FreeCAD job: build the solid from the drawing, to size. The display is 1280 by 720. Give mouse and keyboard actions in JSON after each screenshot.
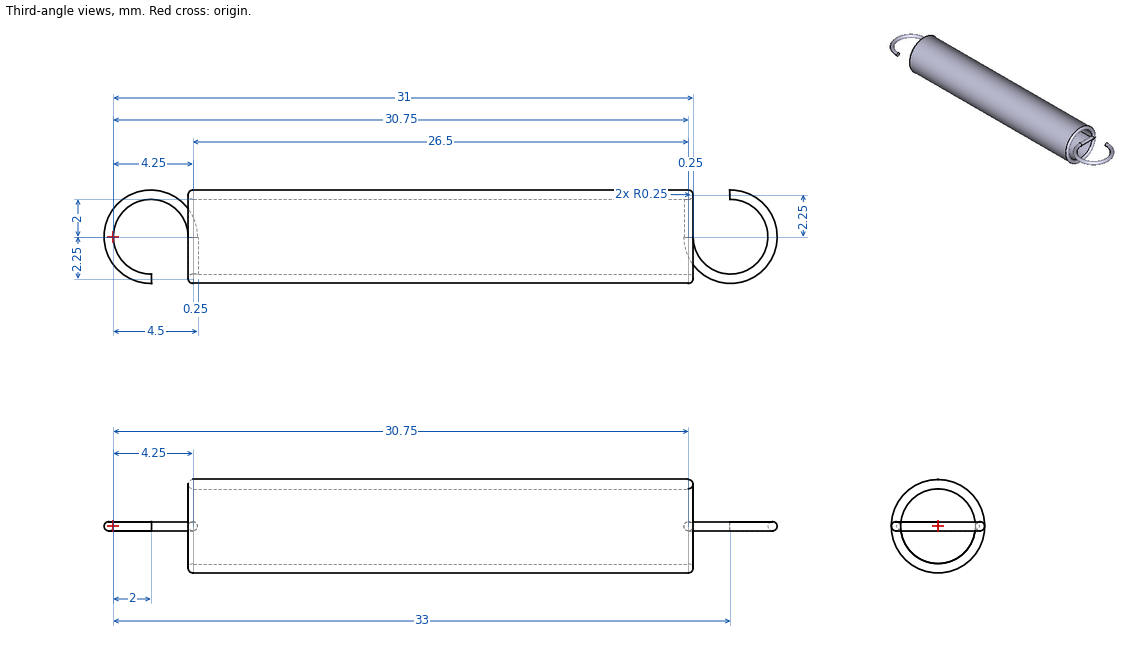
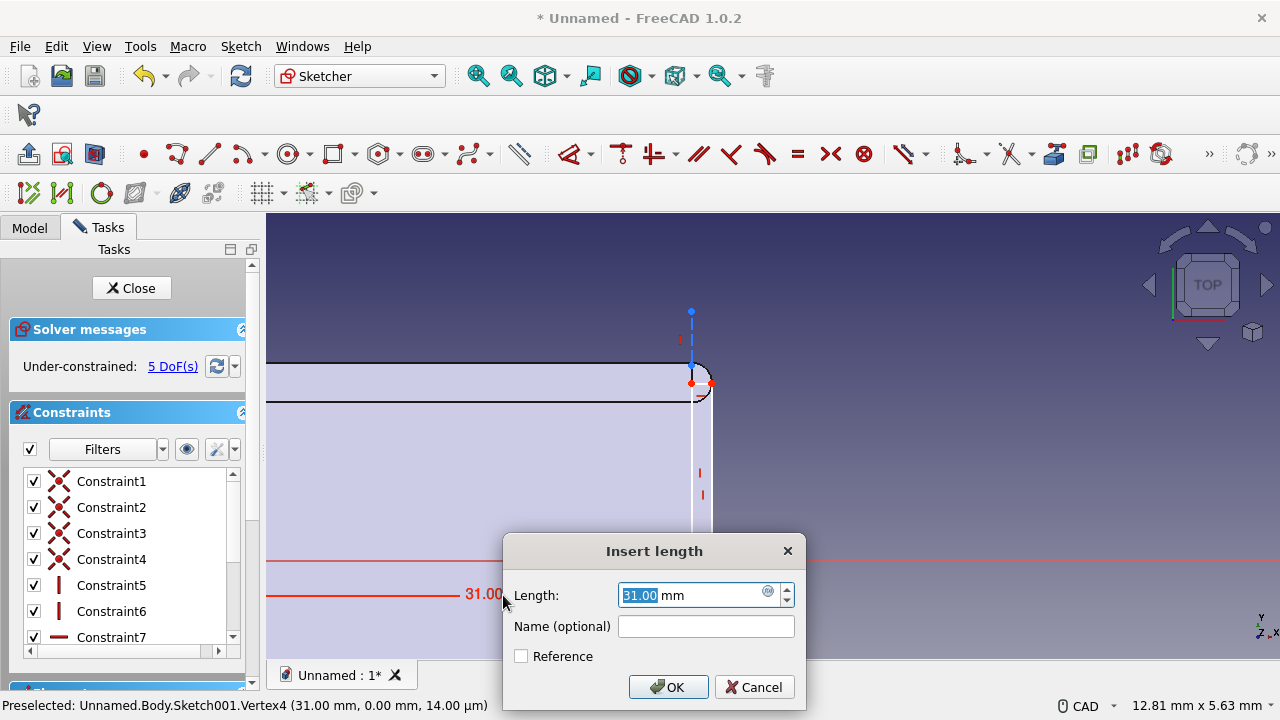
{"action": "type", "text": "31"}
{"action": "key", "text": "Return"}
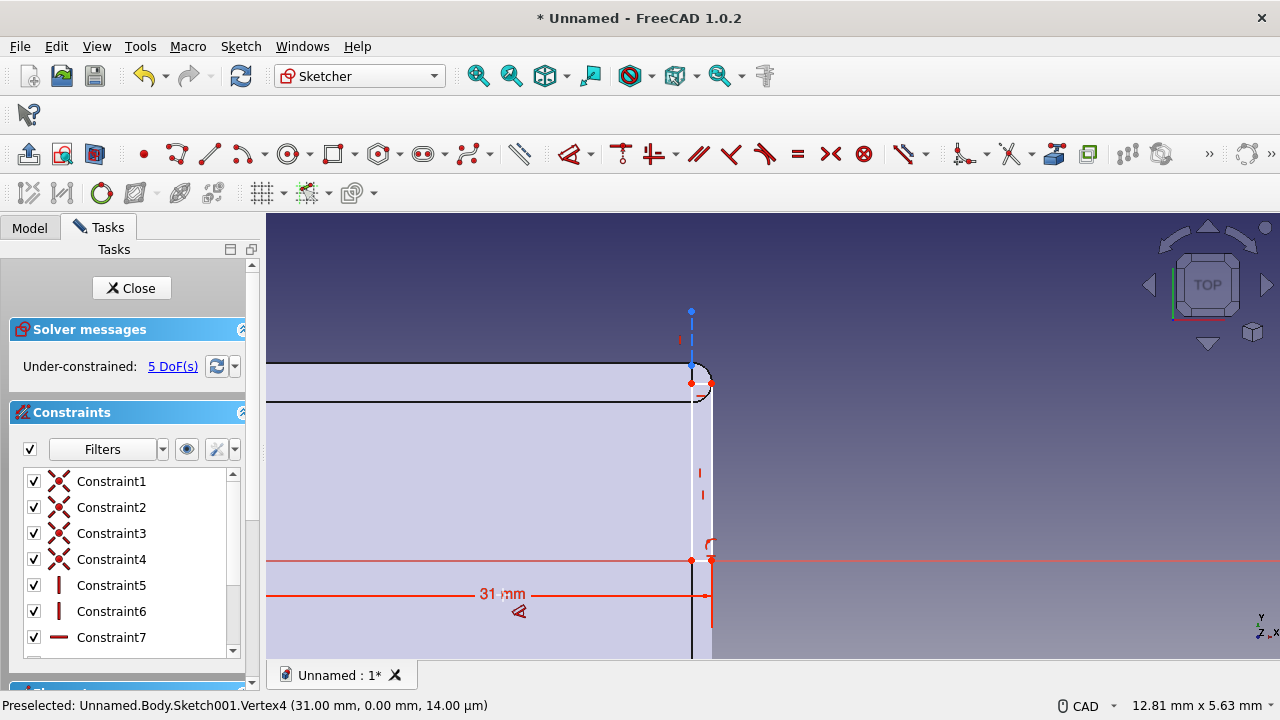
{"action": "left_click", "coordinate": [692, 437]}
{"action": "left_click", "coordinate": [658, 472]}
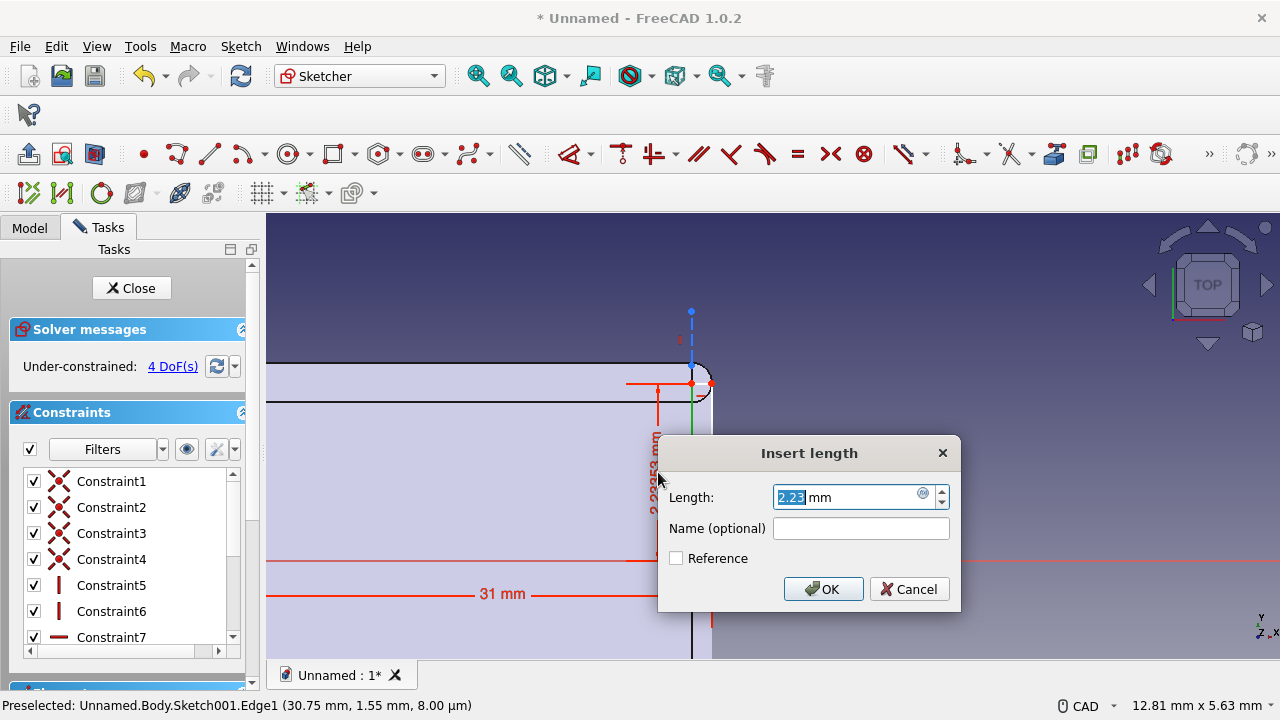
{"action": "type", "text": "2.25"}
{"action": "key", "text": "Return"}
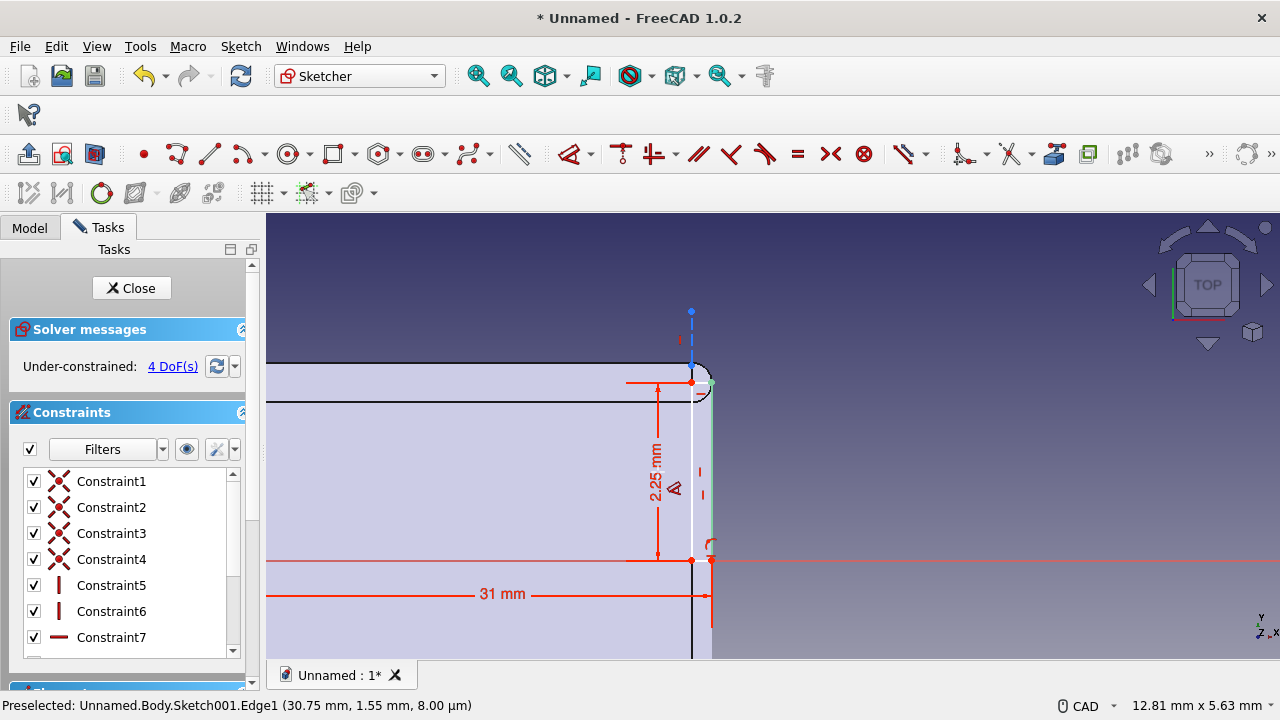
{"action": "scroll", "coordinate": [702, 561], "scroll_direction": "up", "scroll_amount": 4}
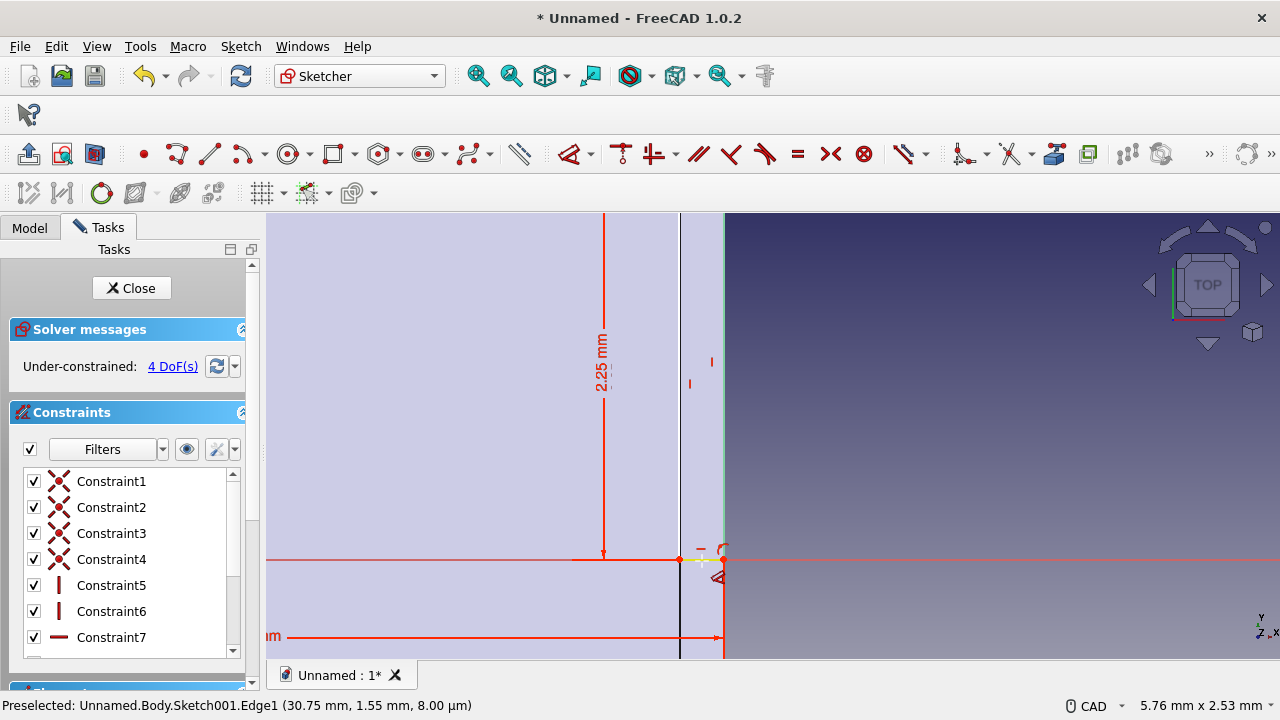
{"action": "left_click", "coordinate": [701, 560]}
{"action": "left_click", "coordinate": [701, 594]}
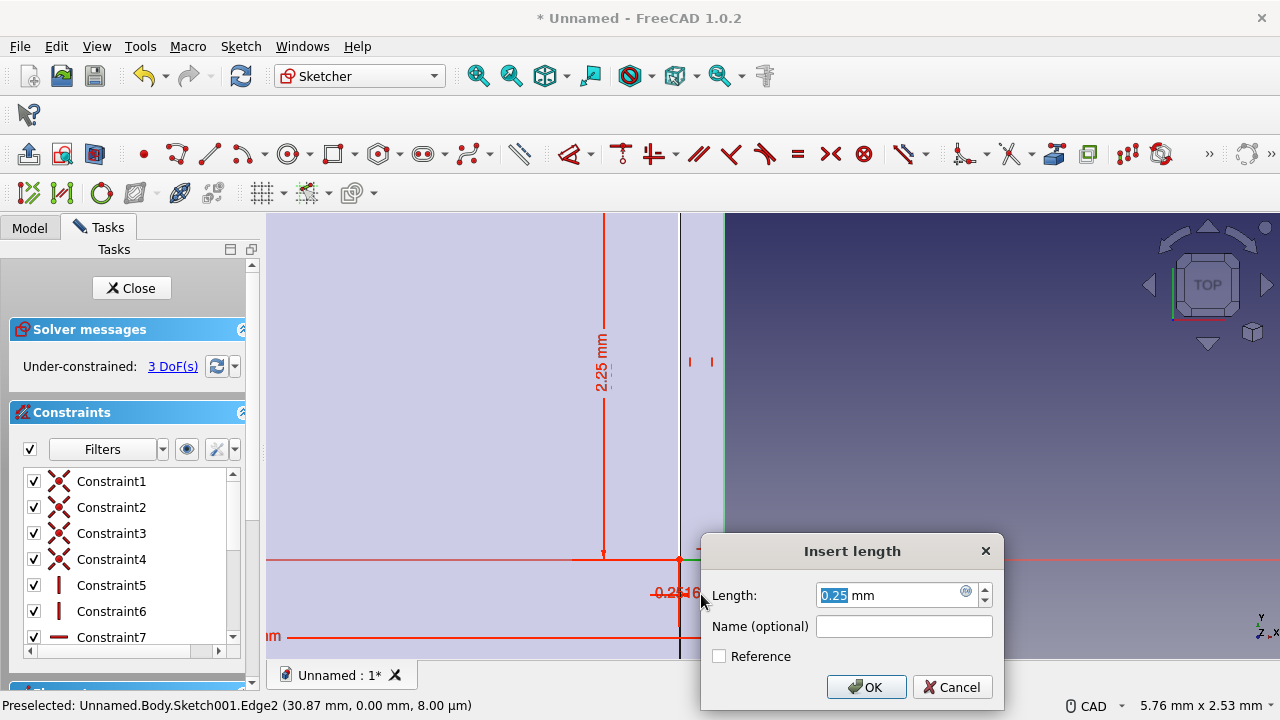
{"action": "type", "text": "0.25"}
{"action": "key", "text": "Return"}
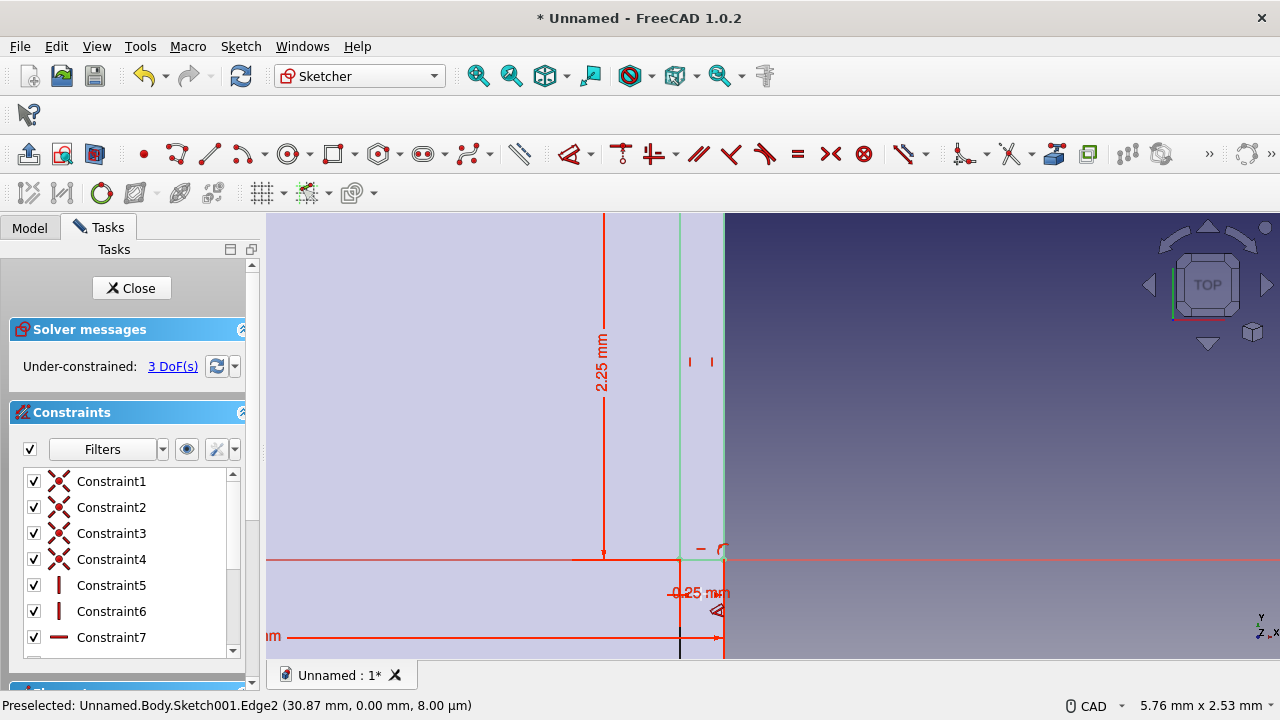
{"action": "scroll", "coordinate": [707, 562], "scroll_direction": "down", "scroll_amount": 4}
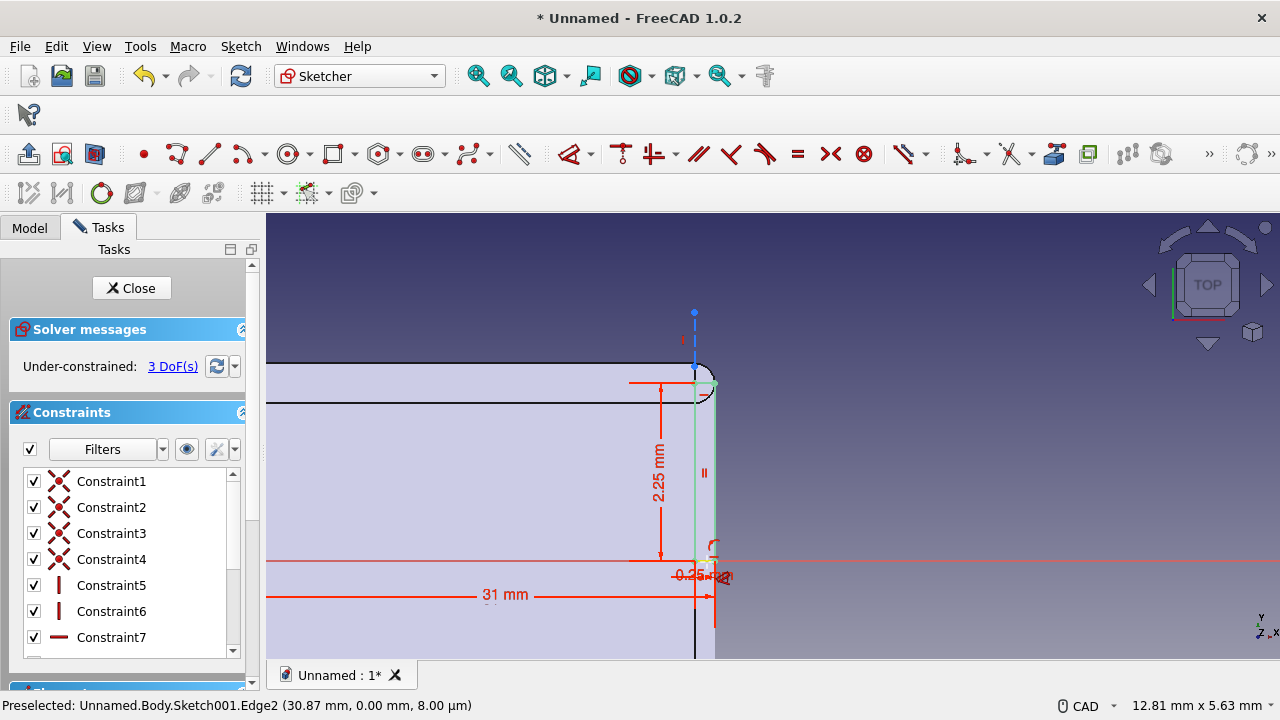
{"action": "left_click", "coordinate": [695, 367]}
{"action": "left_click", "coordinate": [402, 595]}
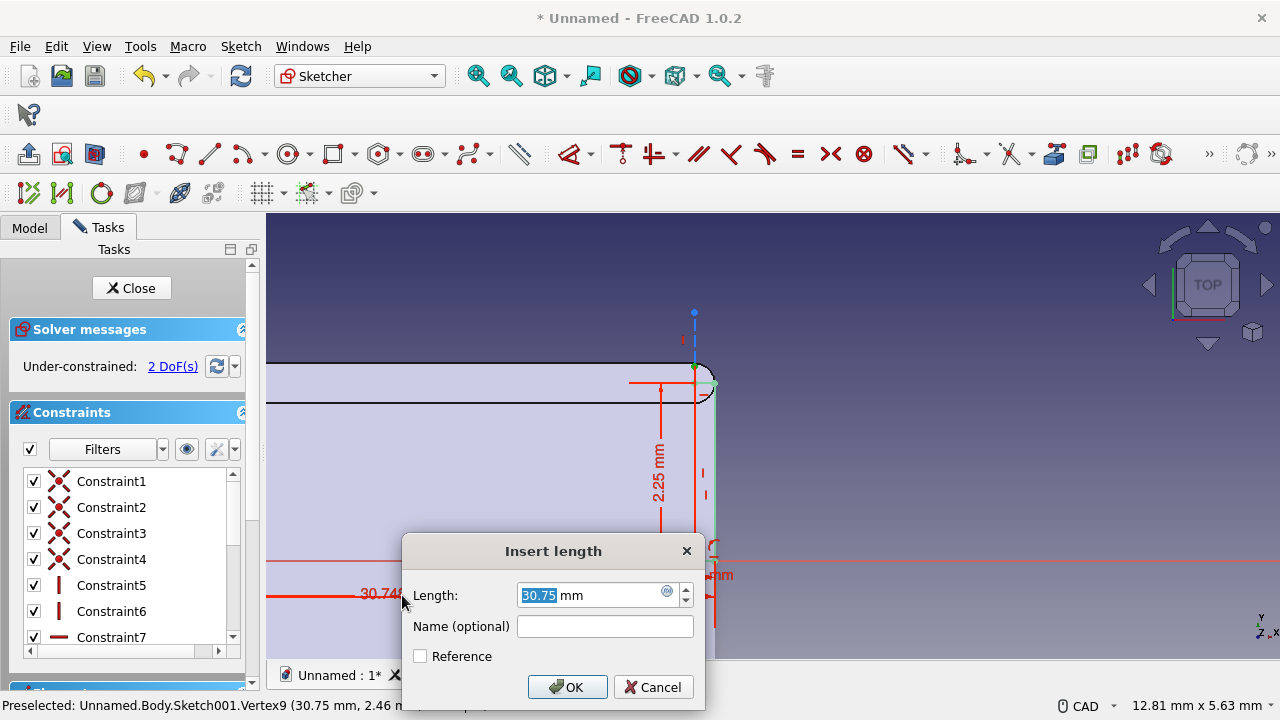
{"action": "type", "text": "30.75"}
{"action": "key", "text": "Return"}
{"action": "key", "text": "Escape"}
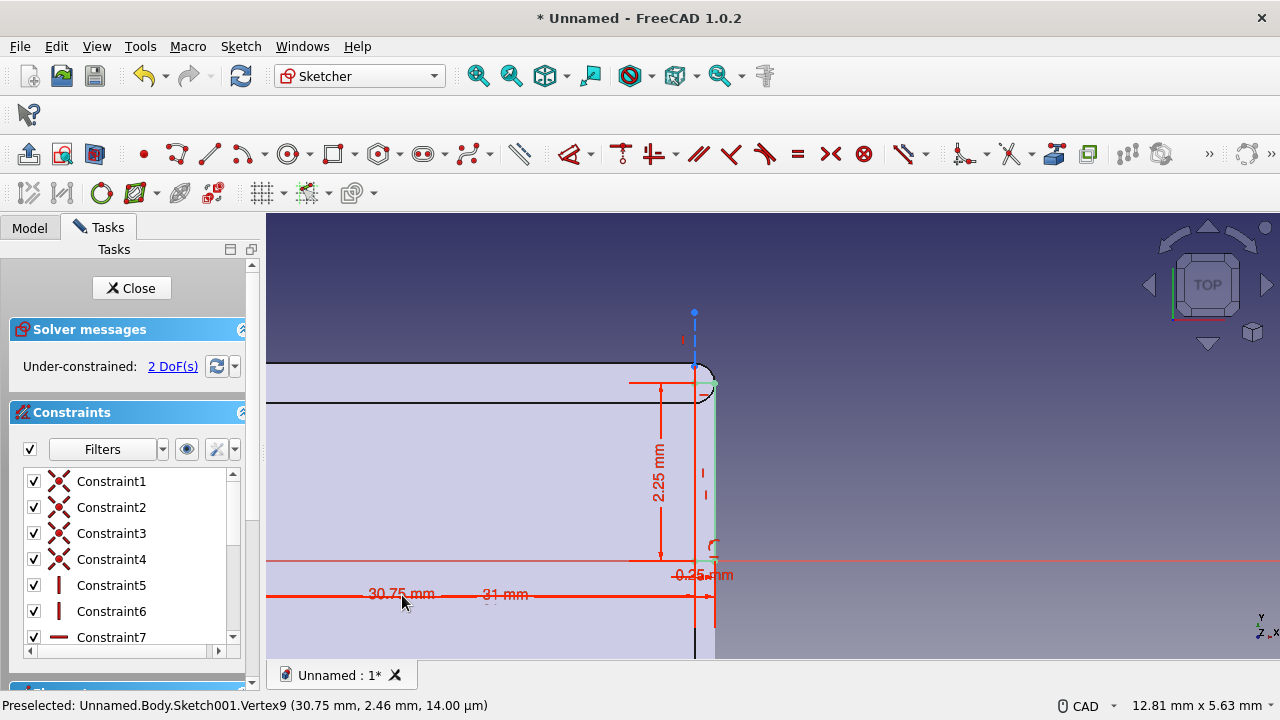
{"action": "left_click", "coordinate": [132, 288]}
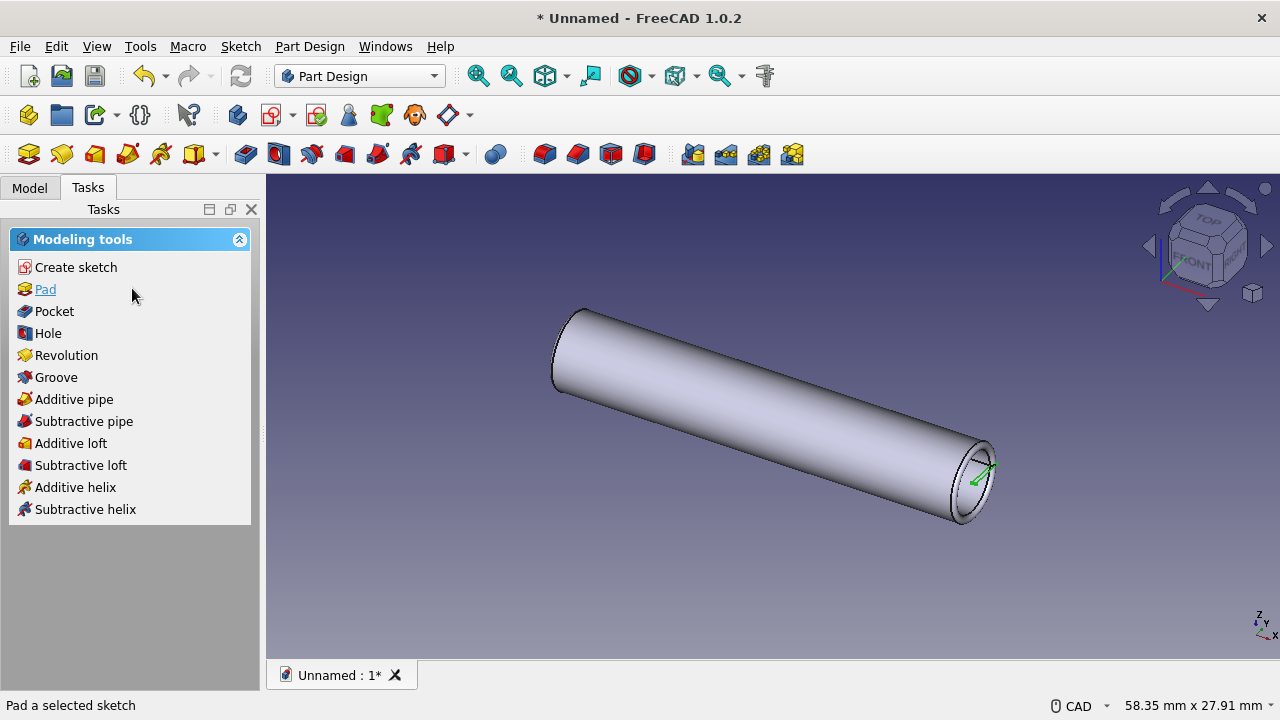
{"action": "left_click", "coordinate": [62, 154]}